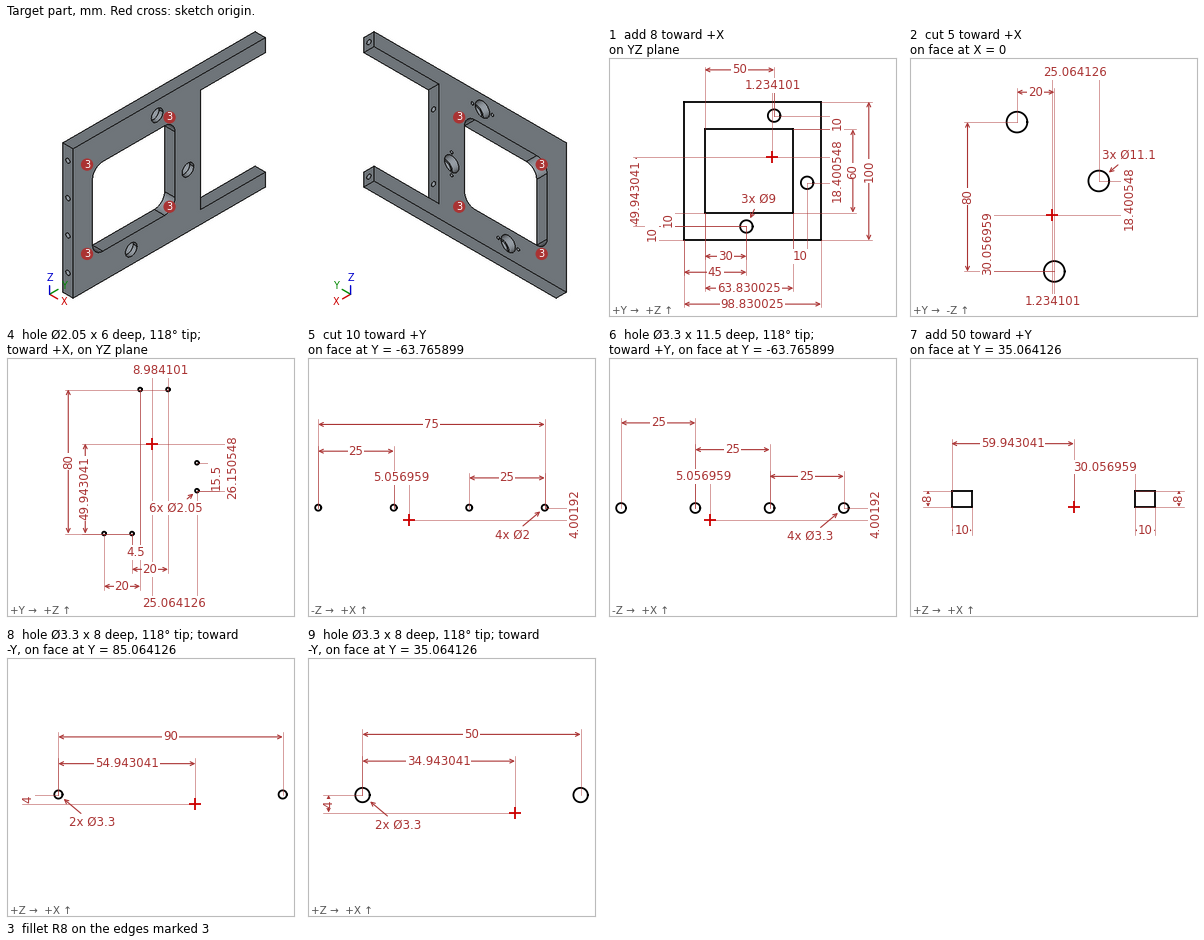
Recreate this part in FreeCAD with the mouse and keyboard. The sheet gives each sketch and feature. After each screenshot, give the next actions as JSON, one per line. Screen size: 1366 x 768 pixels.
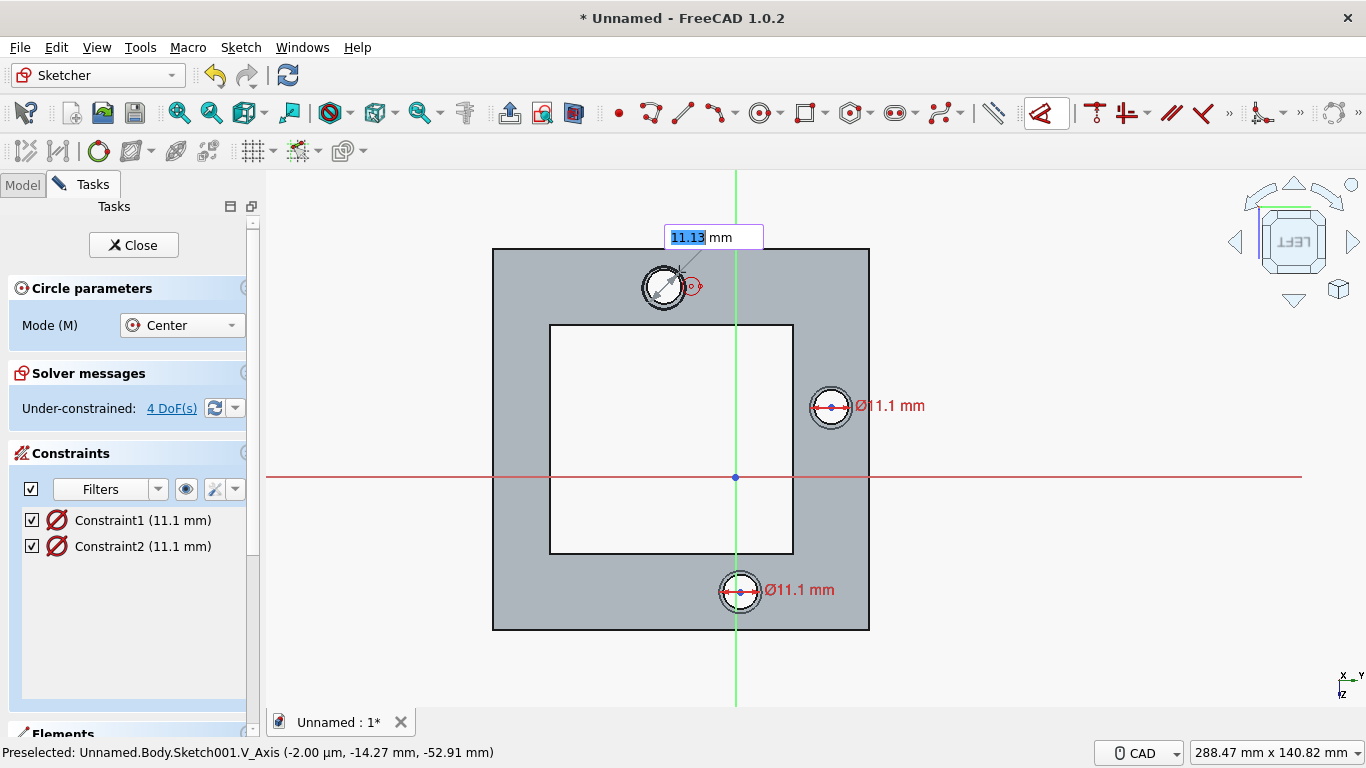
{"action": "type", "text": "11.1"}
{"action": "key", "text": "Return"}
{"action": "key", "text": "Escape"}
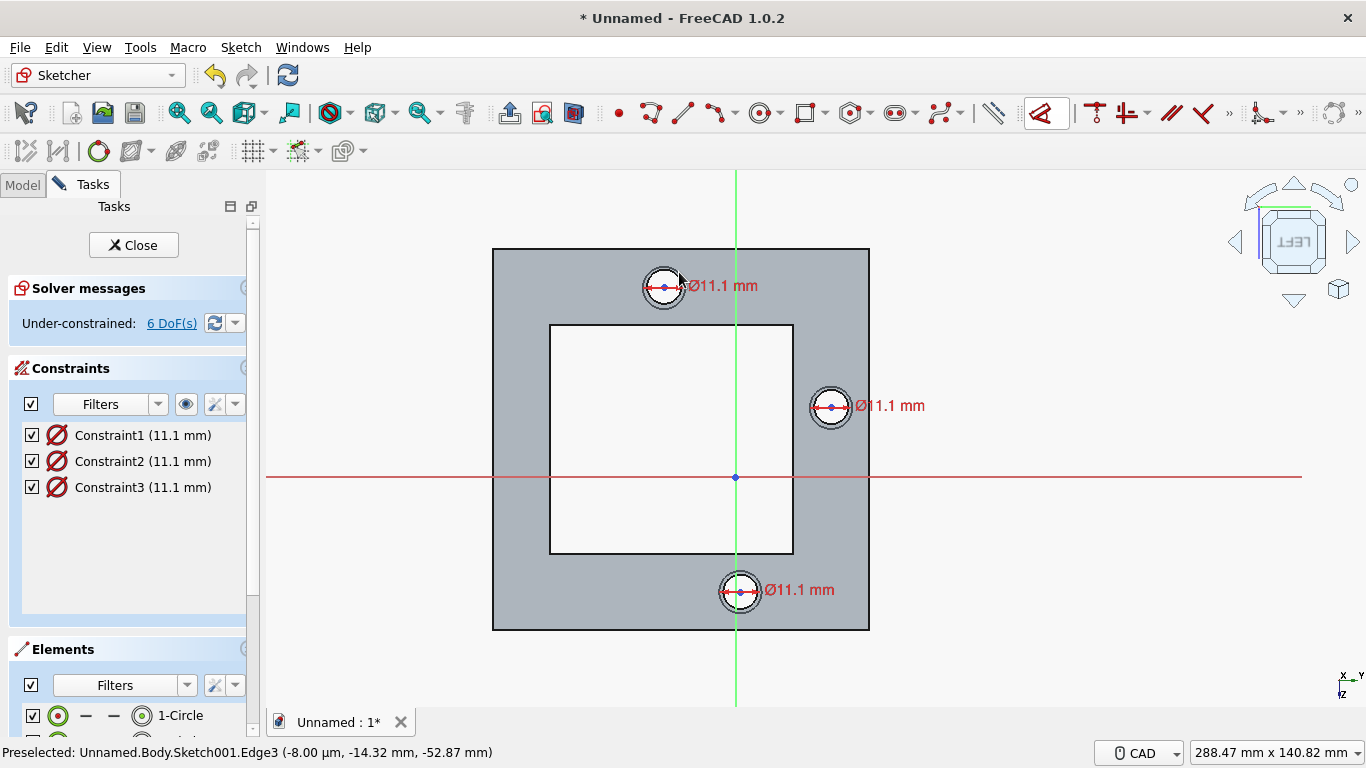
{"action": "left_click", "coordinate": [740, 592]}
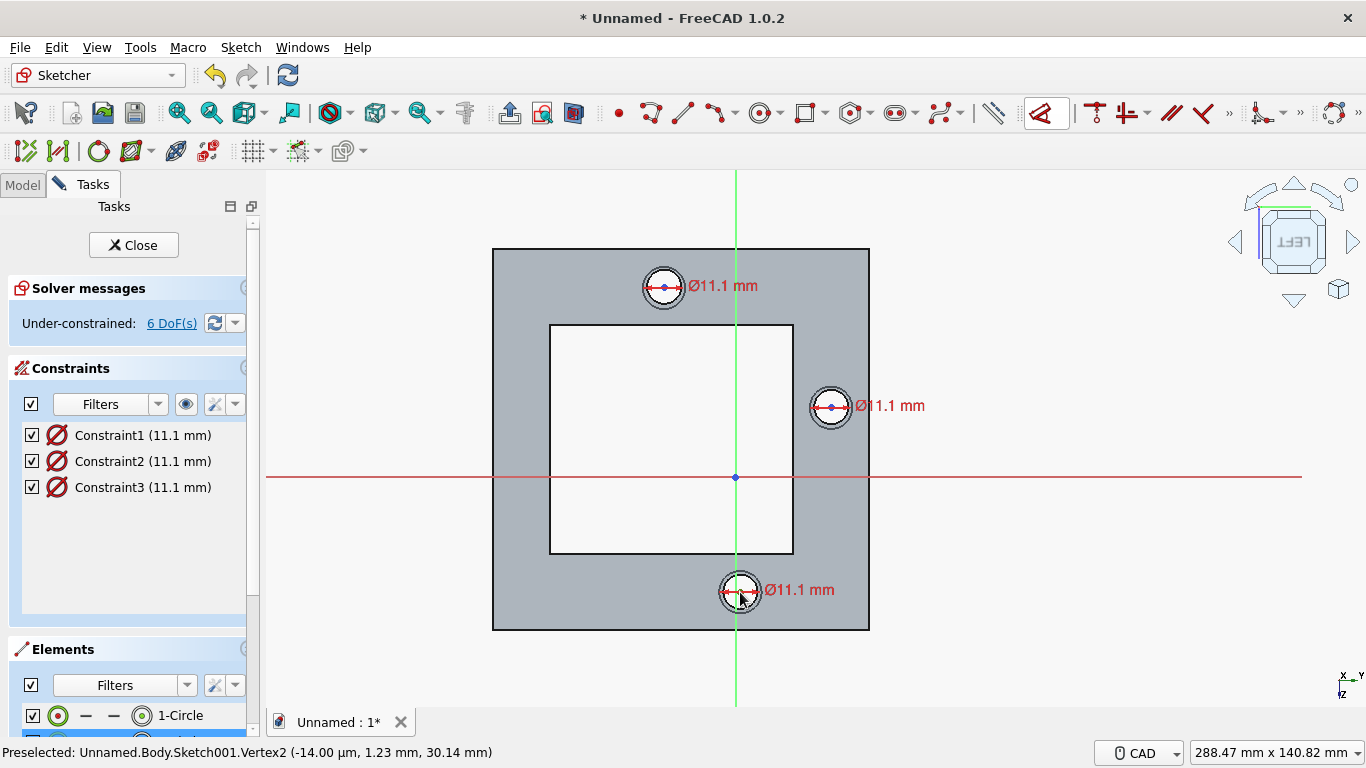
{"action": "left_click", "coordinate": [664, 288]}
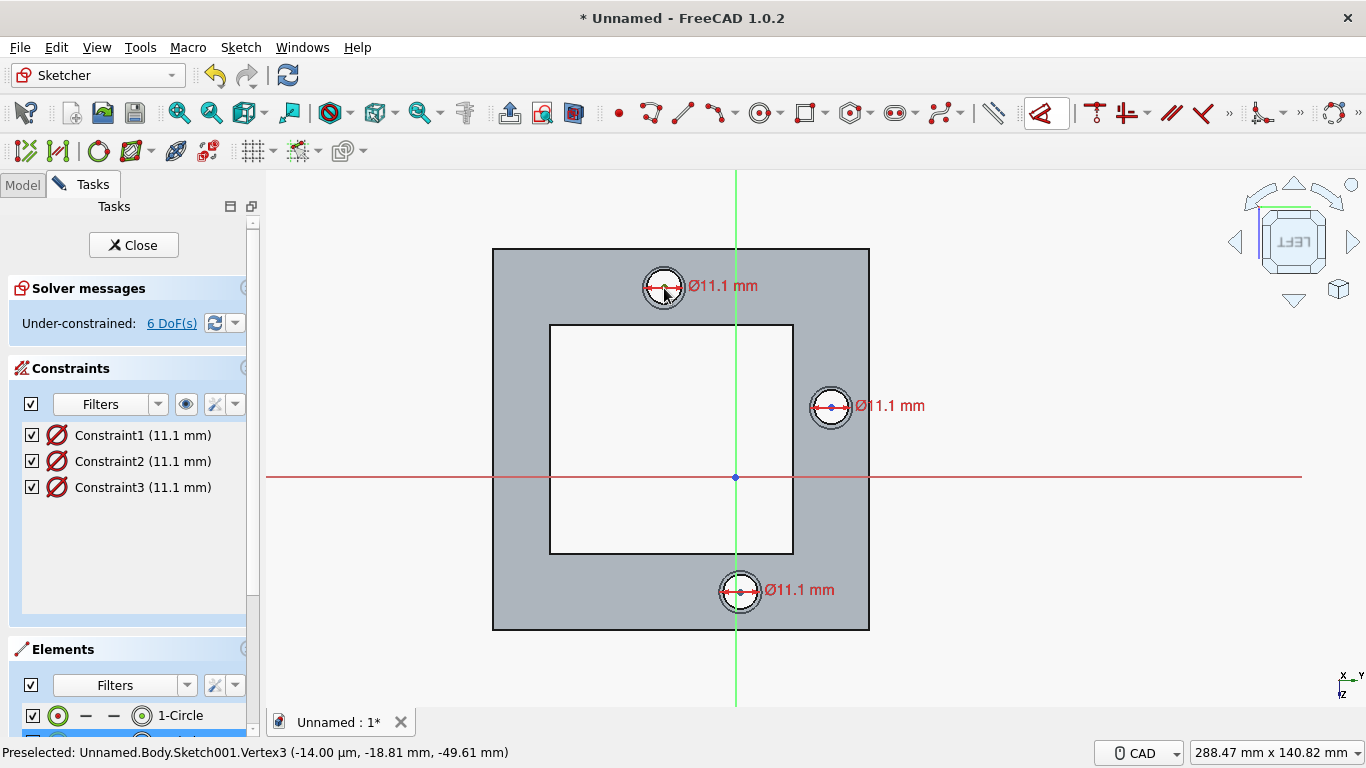
{"action": "left_click", "coordinate": [1064, 114]}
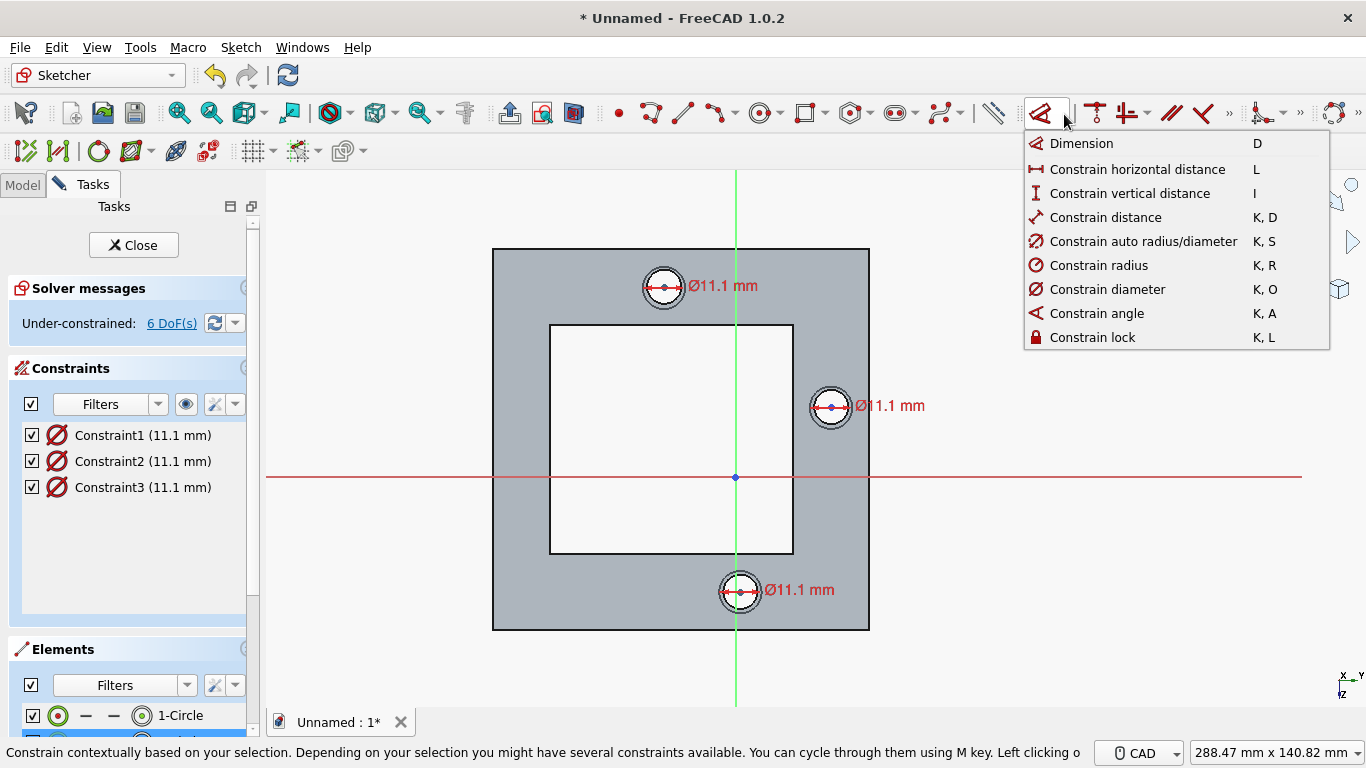
{"action": "left_click", "coordinate": [1177, 169]}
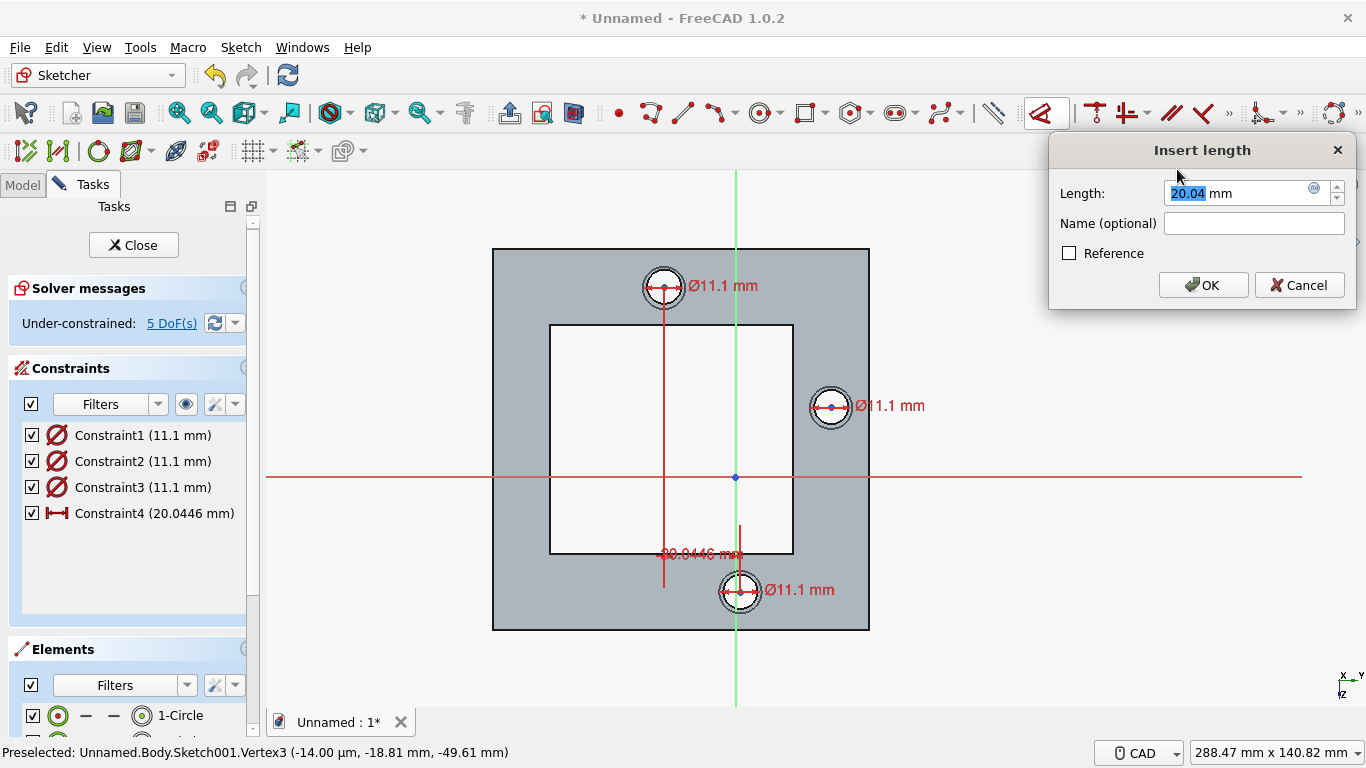
{"action": "type", "text": "20"}
{"action": "key", "text": "Return"}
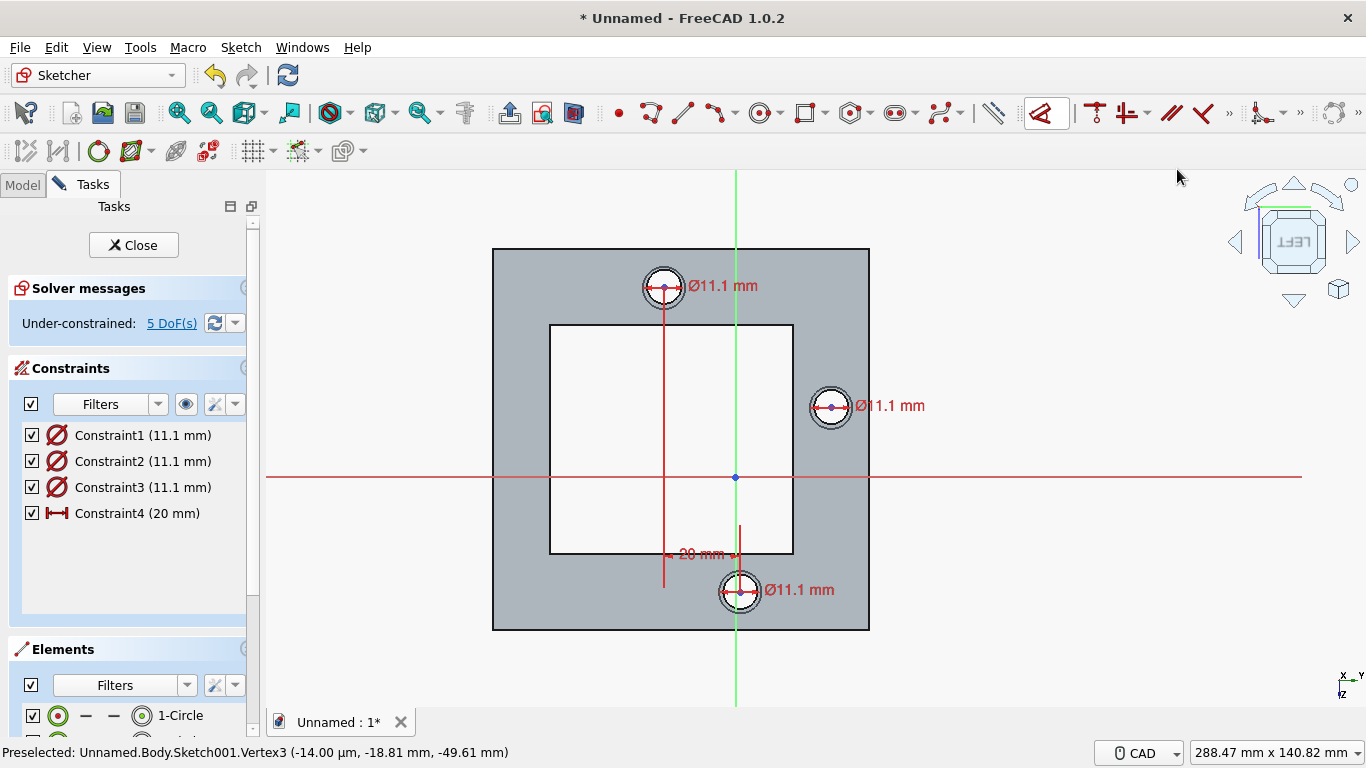
{"action": "left_click", "coordinate": [740, 592]}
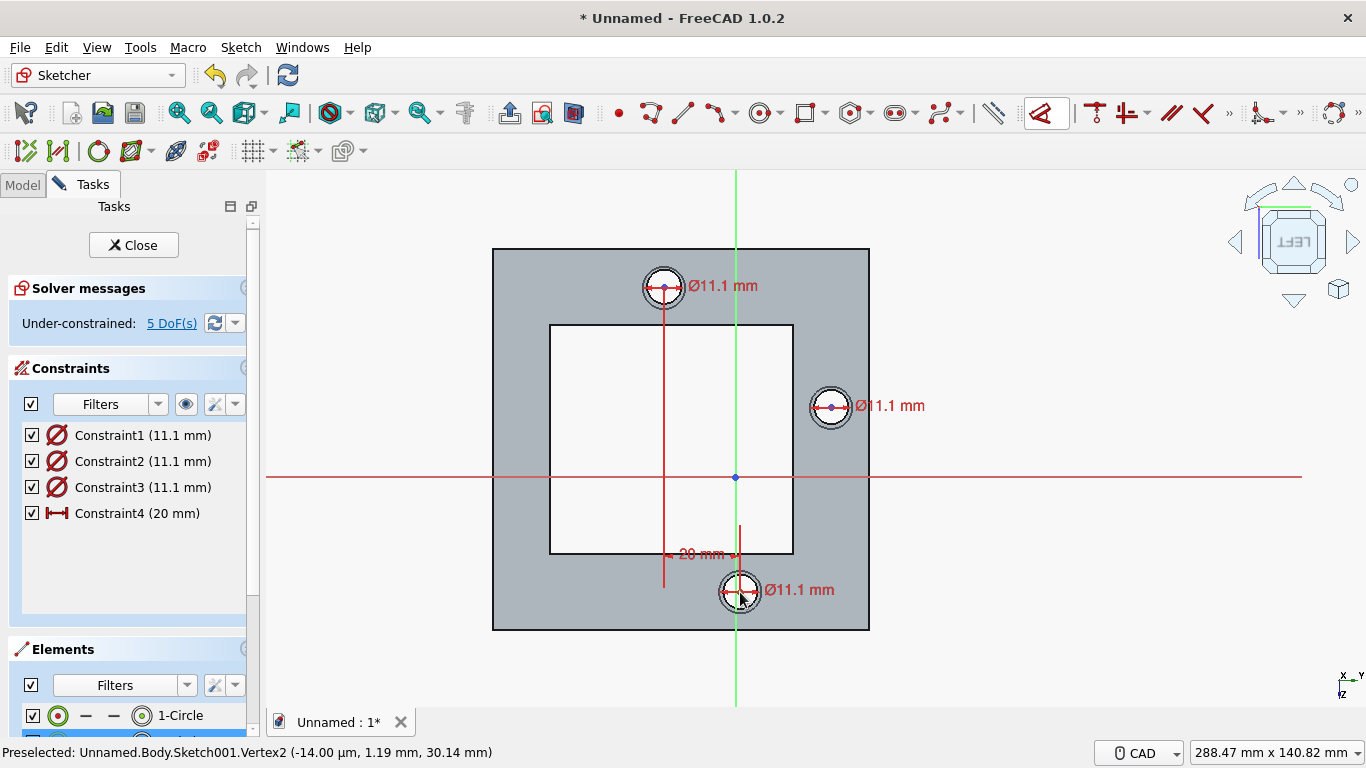
{"action": "left_click", "coordinate": [664, 288]}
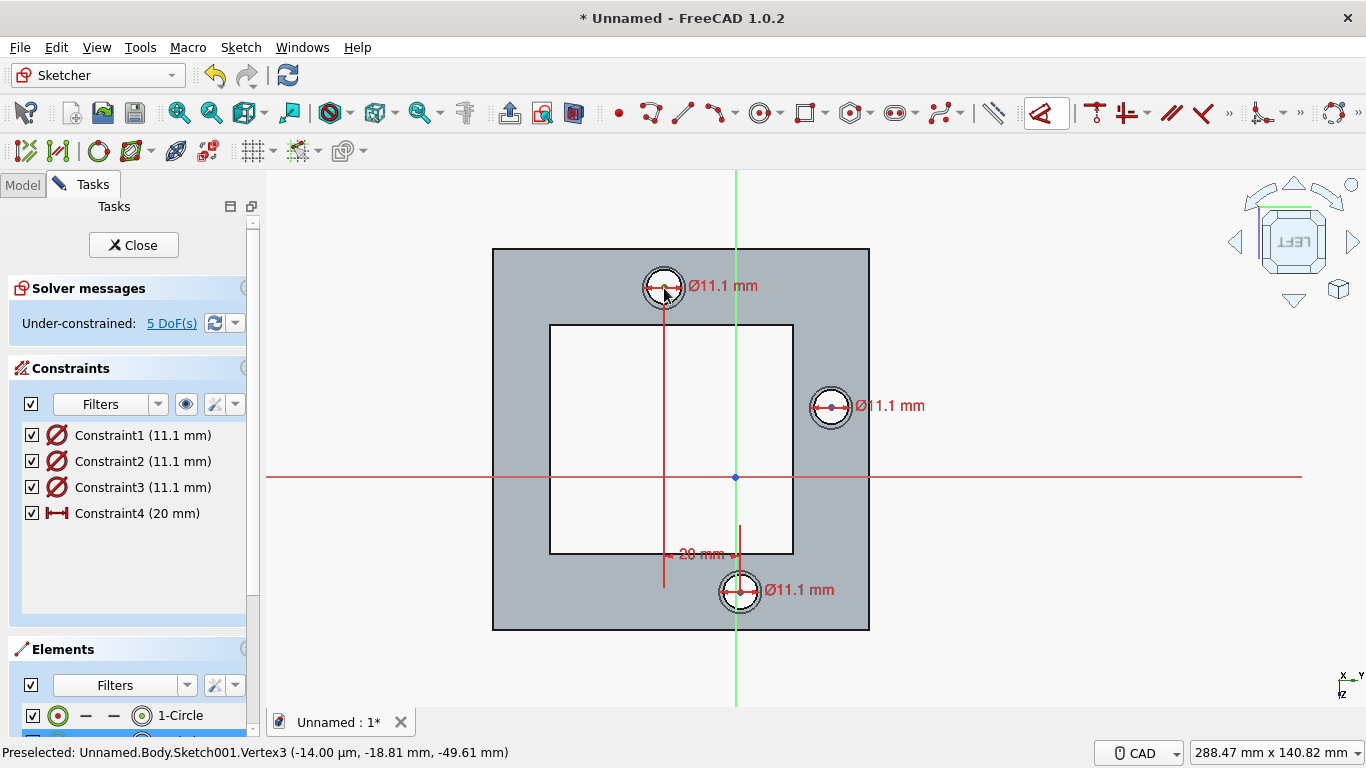
{"action": "key", "text": "i"}